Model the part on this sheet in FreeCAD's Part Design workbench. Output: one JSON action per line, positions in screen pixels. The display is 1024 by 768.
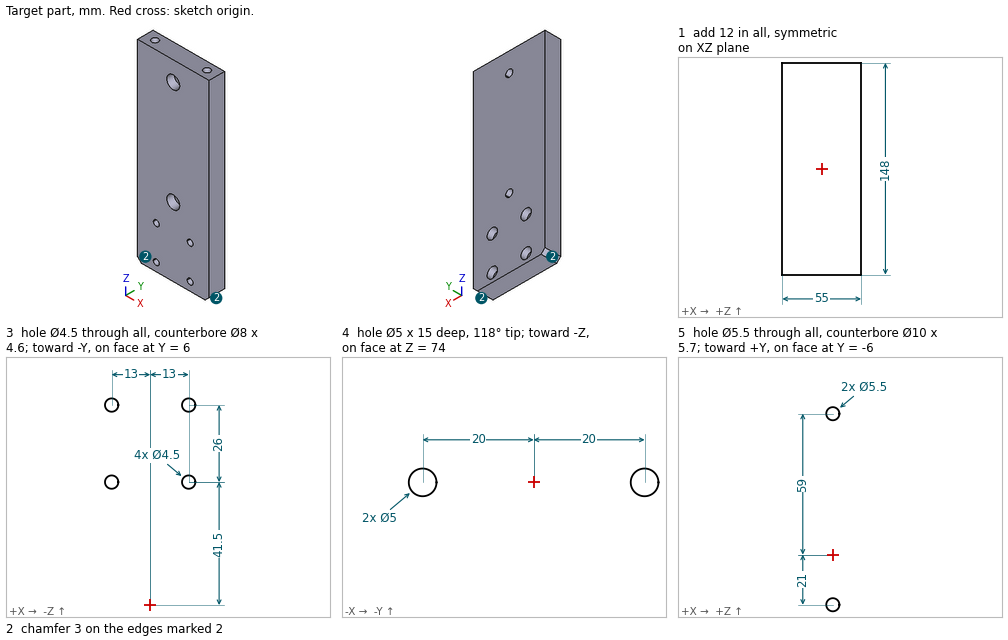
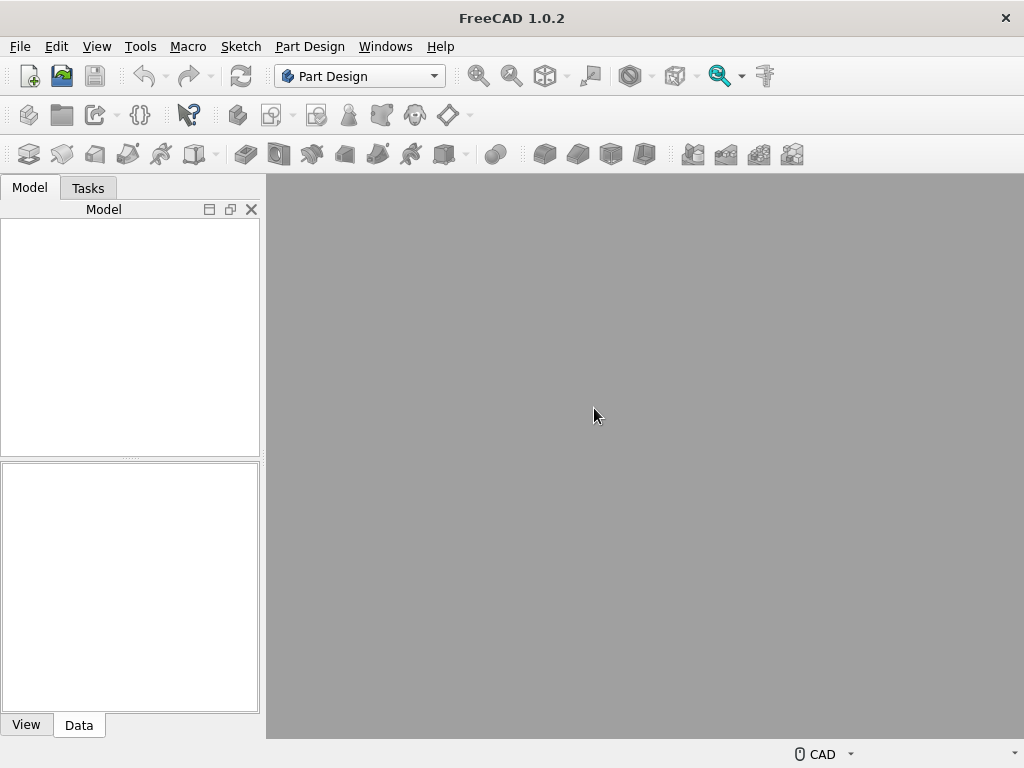
{"action": "left_click", "coordinate": [29, 76]}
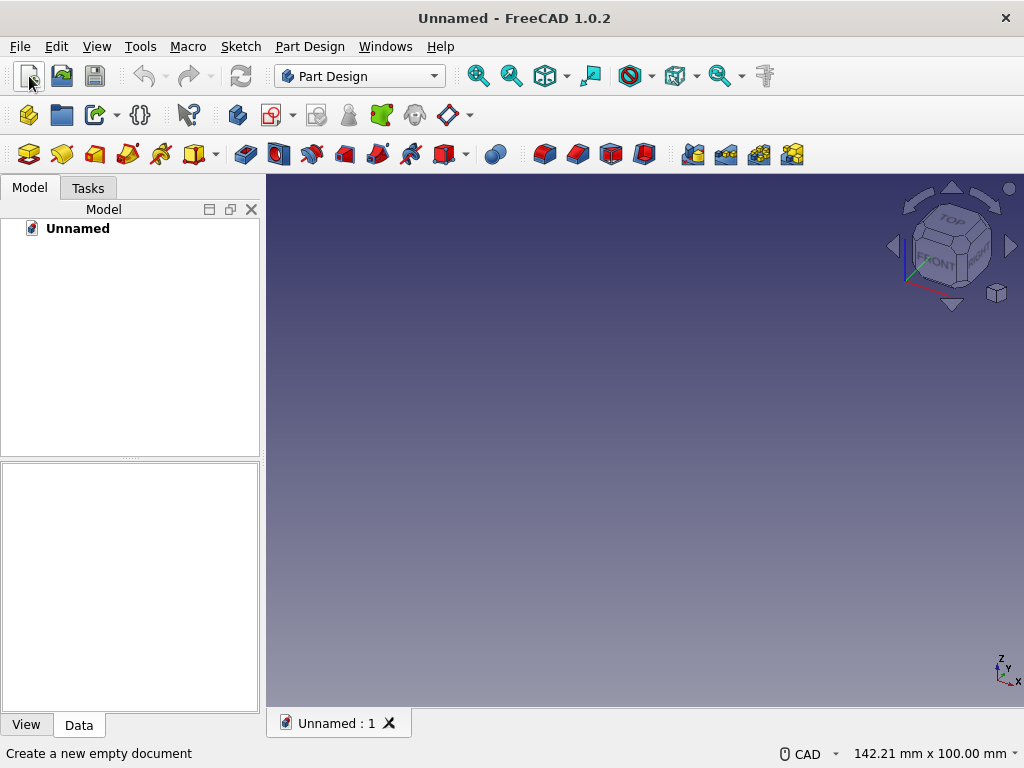
{"action": "left_click", "coordinate": [270, 116]}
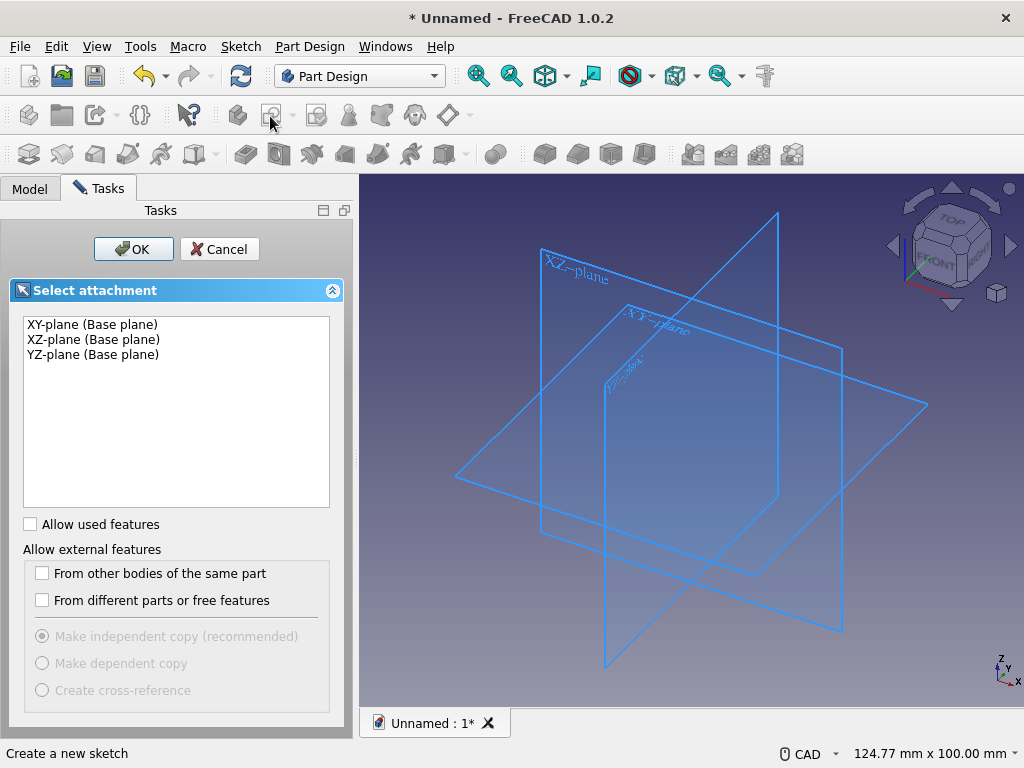
{"action": "left_click", "coordinate": [84, 340]}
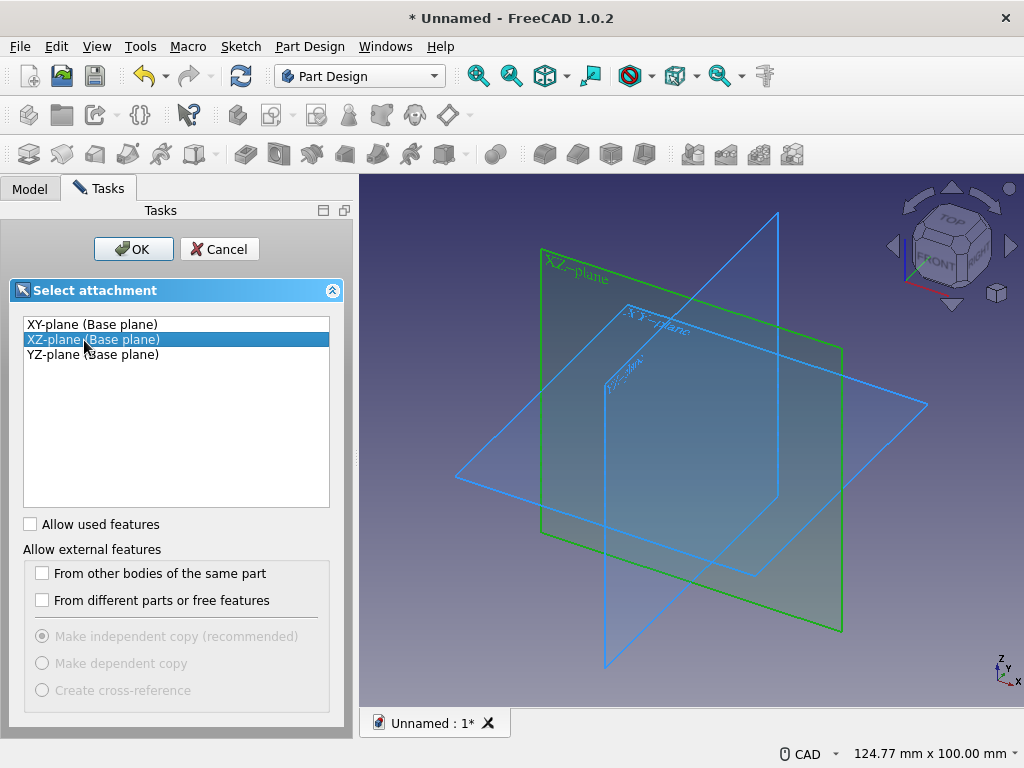
{"action": "left_click", "coordinate": [134, 249]}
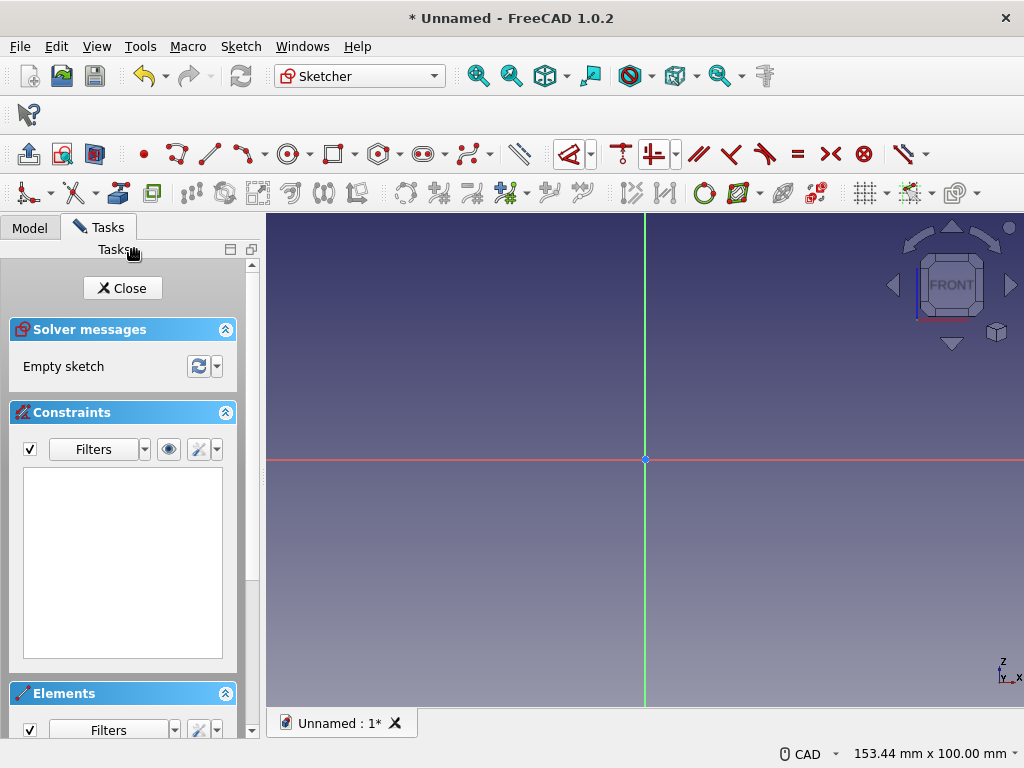
{"action": "scroll", "coordinate": [521, 460], "scroll_direction": "down", "scroll_amount": 4}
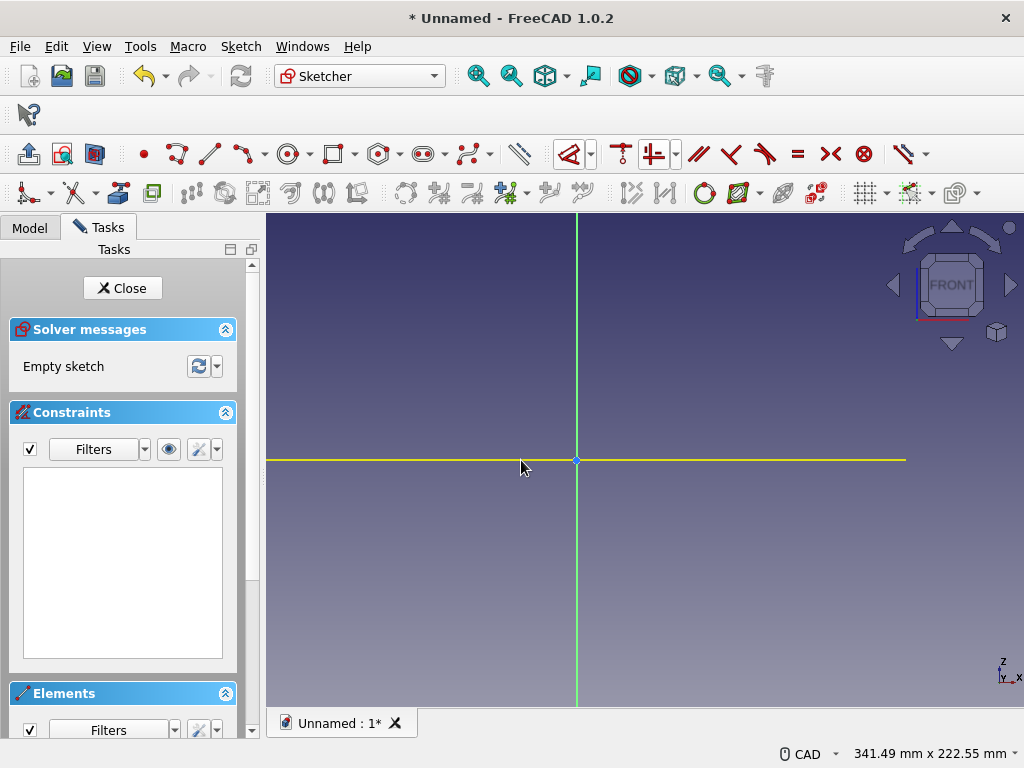
{"action": "key", "text": "g v"}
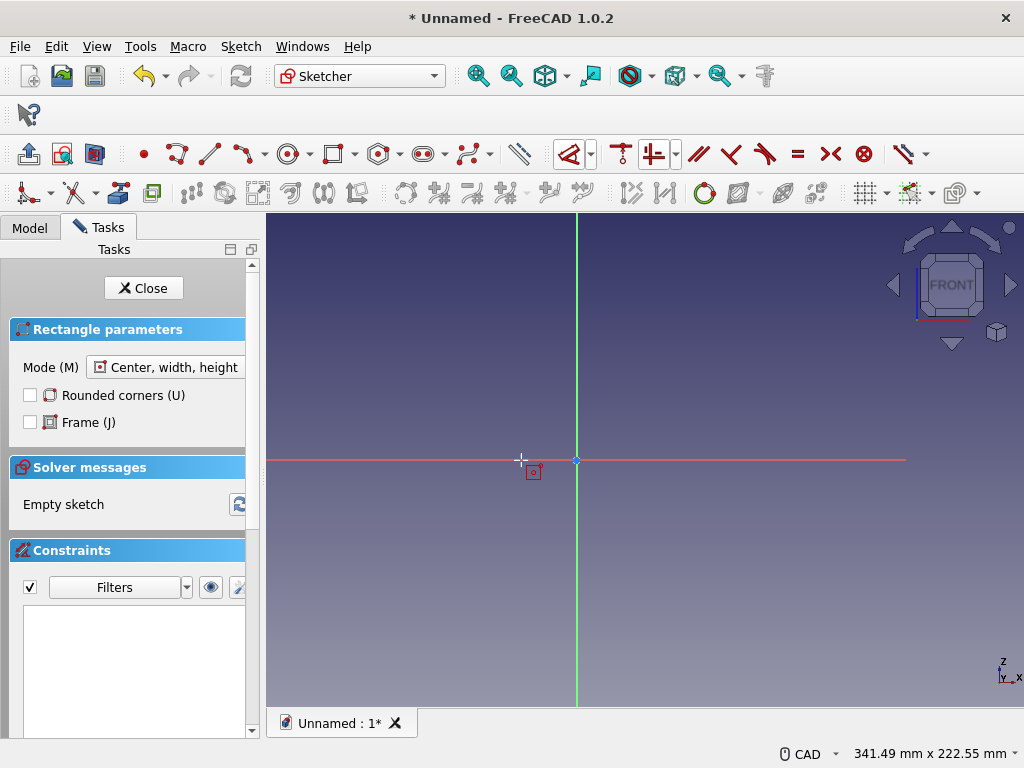
{"action": "left_click", "coordinate": [577, 460]}
{"action": "mouse_move", "coordinate": [638, 296]}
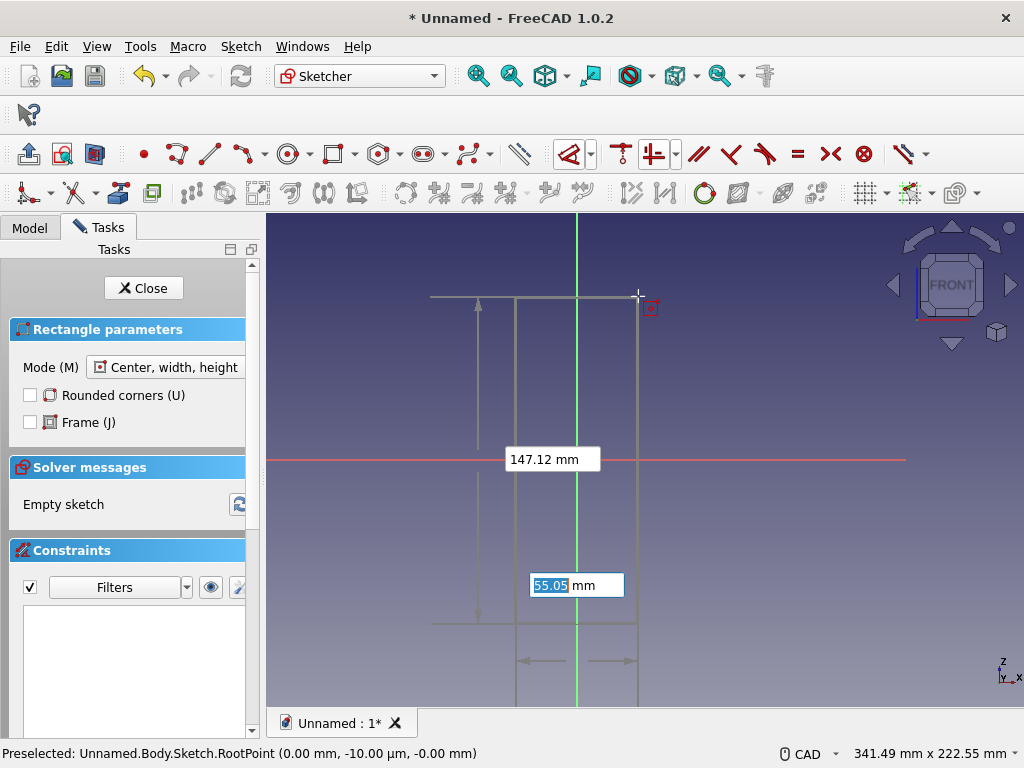
{"action": "type", "text": "55"}
{"action": "key", "text": "Tab"}
{"action": "type", "text": "148"}
{"action": "key", "text": "Return"}
{"action": "key", "text": "Escape"}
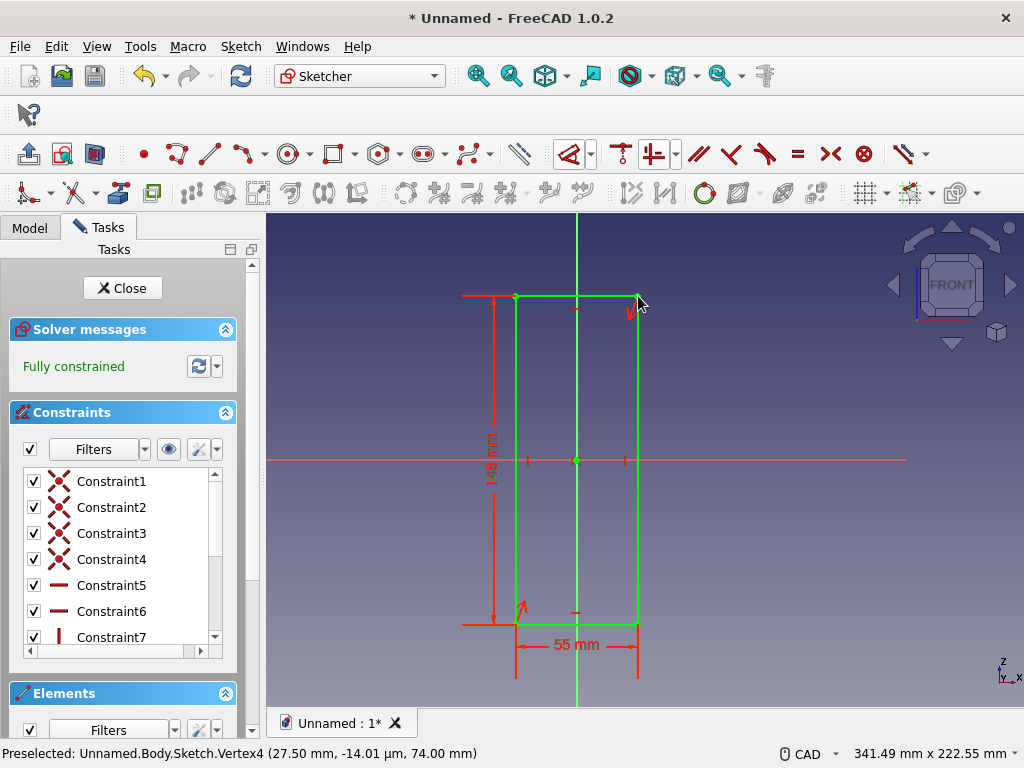
{"action": "left_click", "coordinate": [123, 288]}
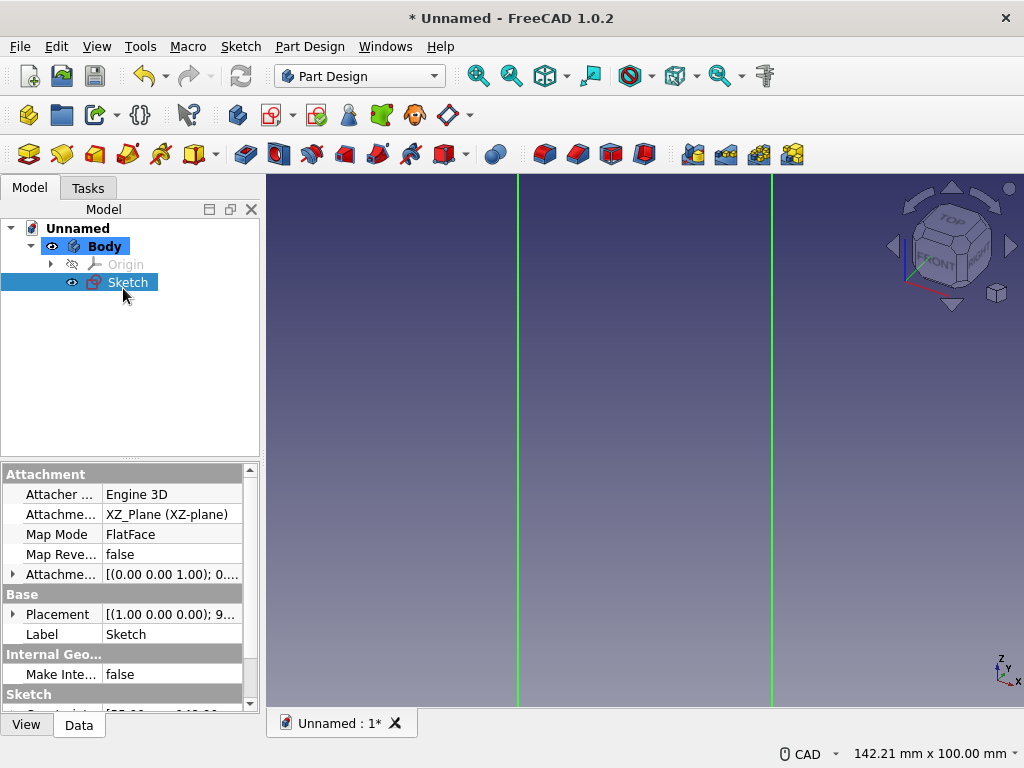
{"action": "left_click", "coordinate": [29, 154]}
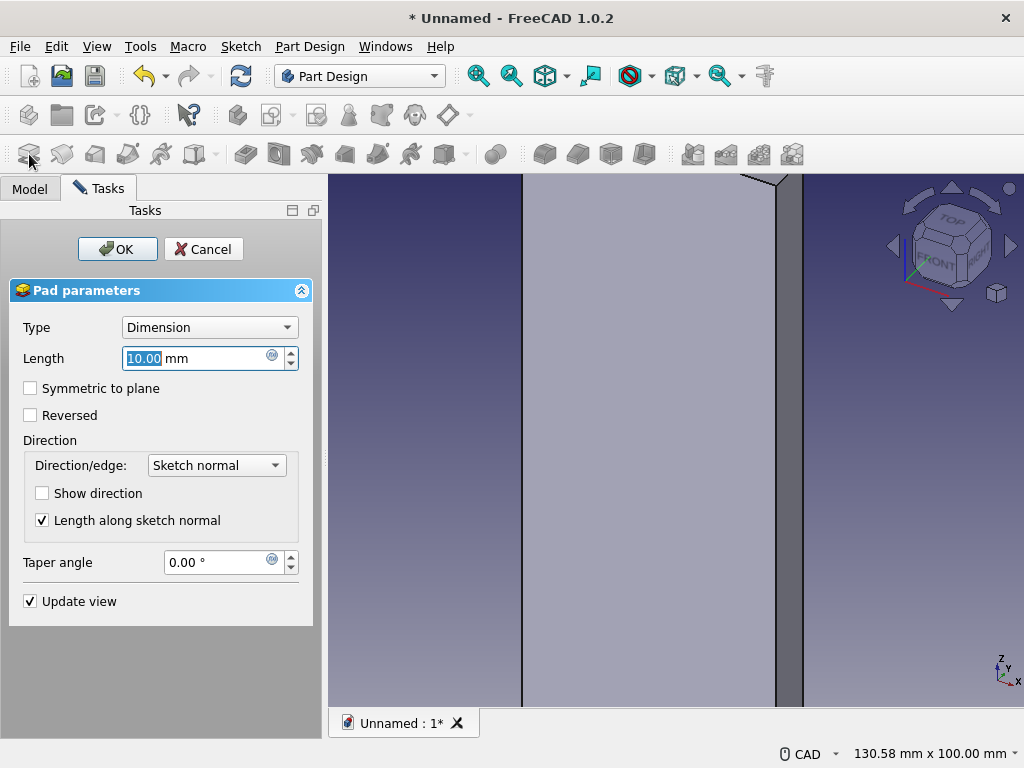
{"action": "type", "text": "12"}
{"action": "key", "text": "Tab"}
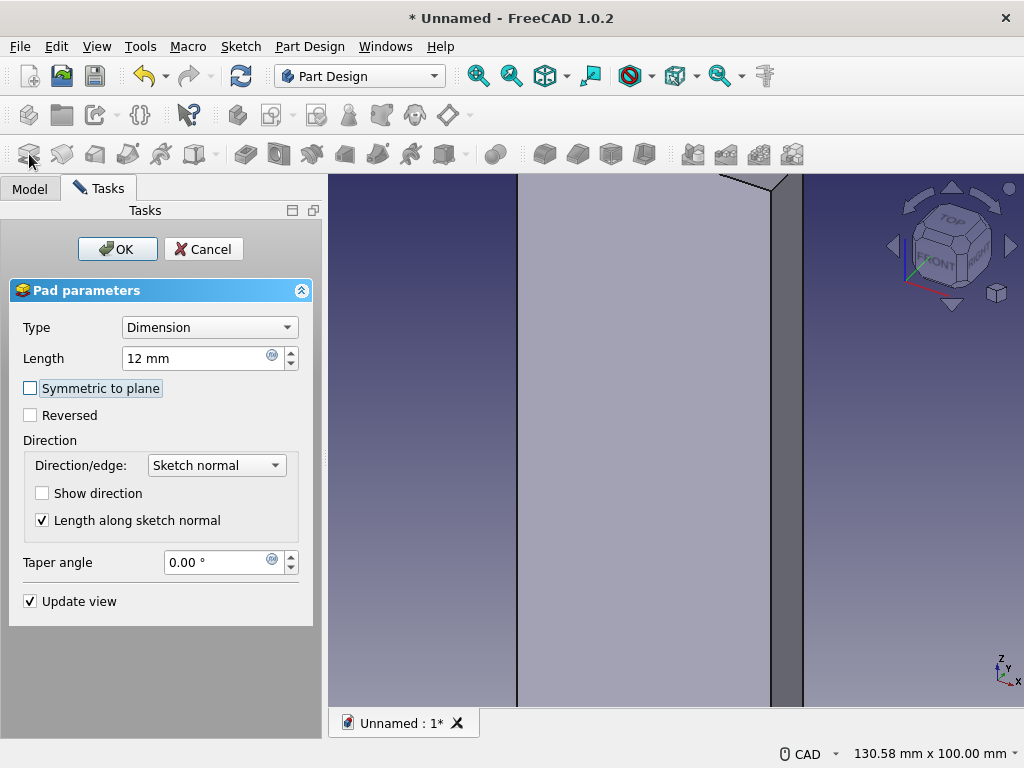
{"action": "left_click", "coordinate": [31, 388]}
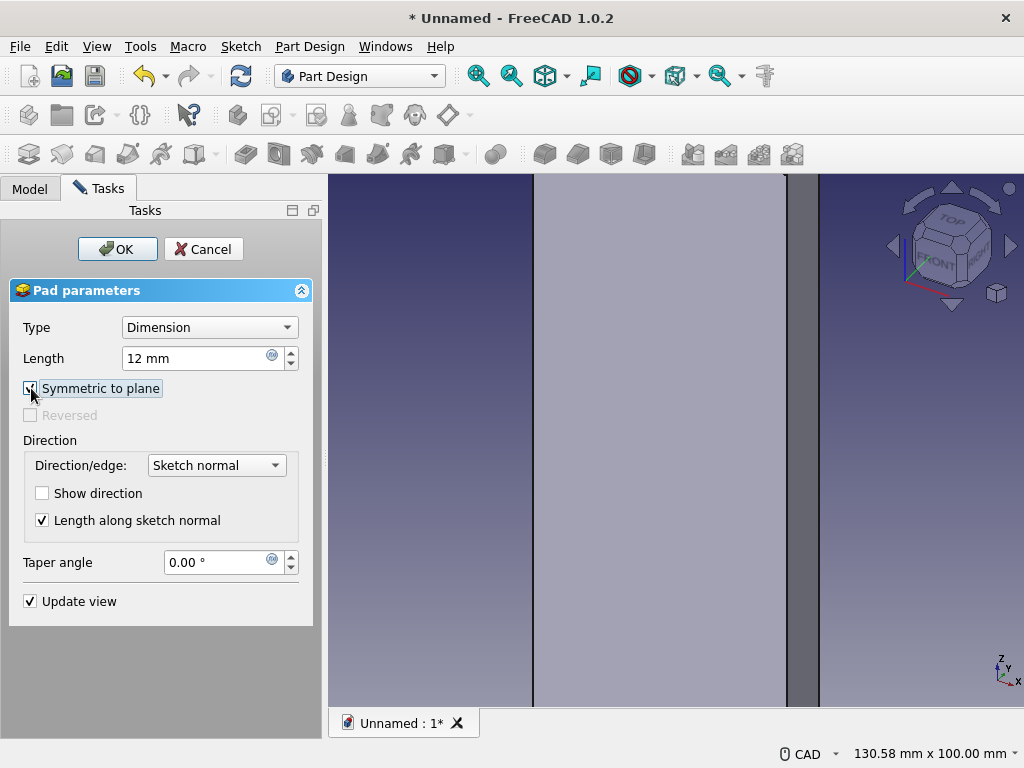
{"action": "left_click", "coordinate": [118, 249]}